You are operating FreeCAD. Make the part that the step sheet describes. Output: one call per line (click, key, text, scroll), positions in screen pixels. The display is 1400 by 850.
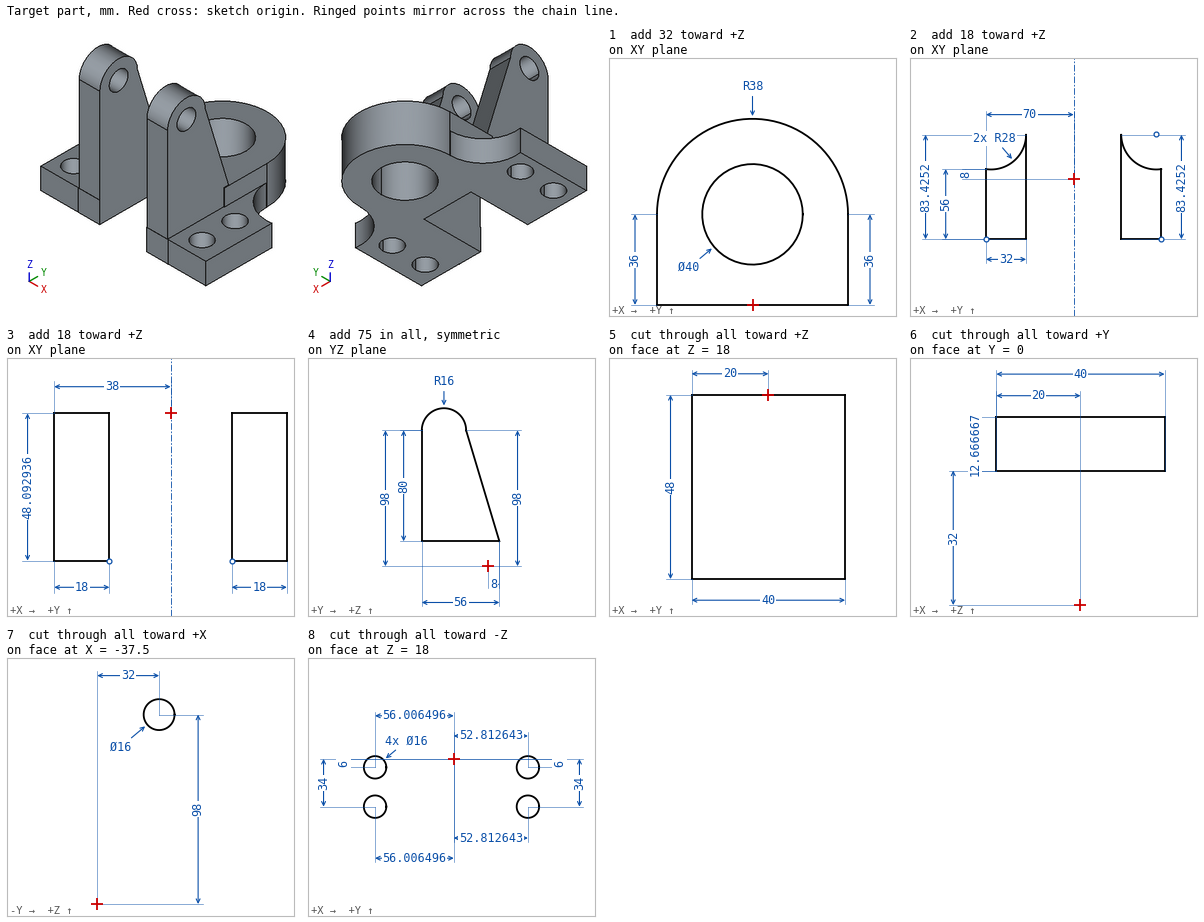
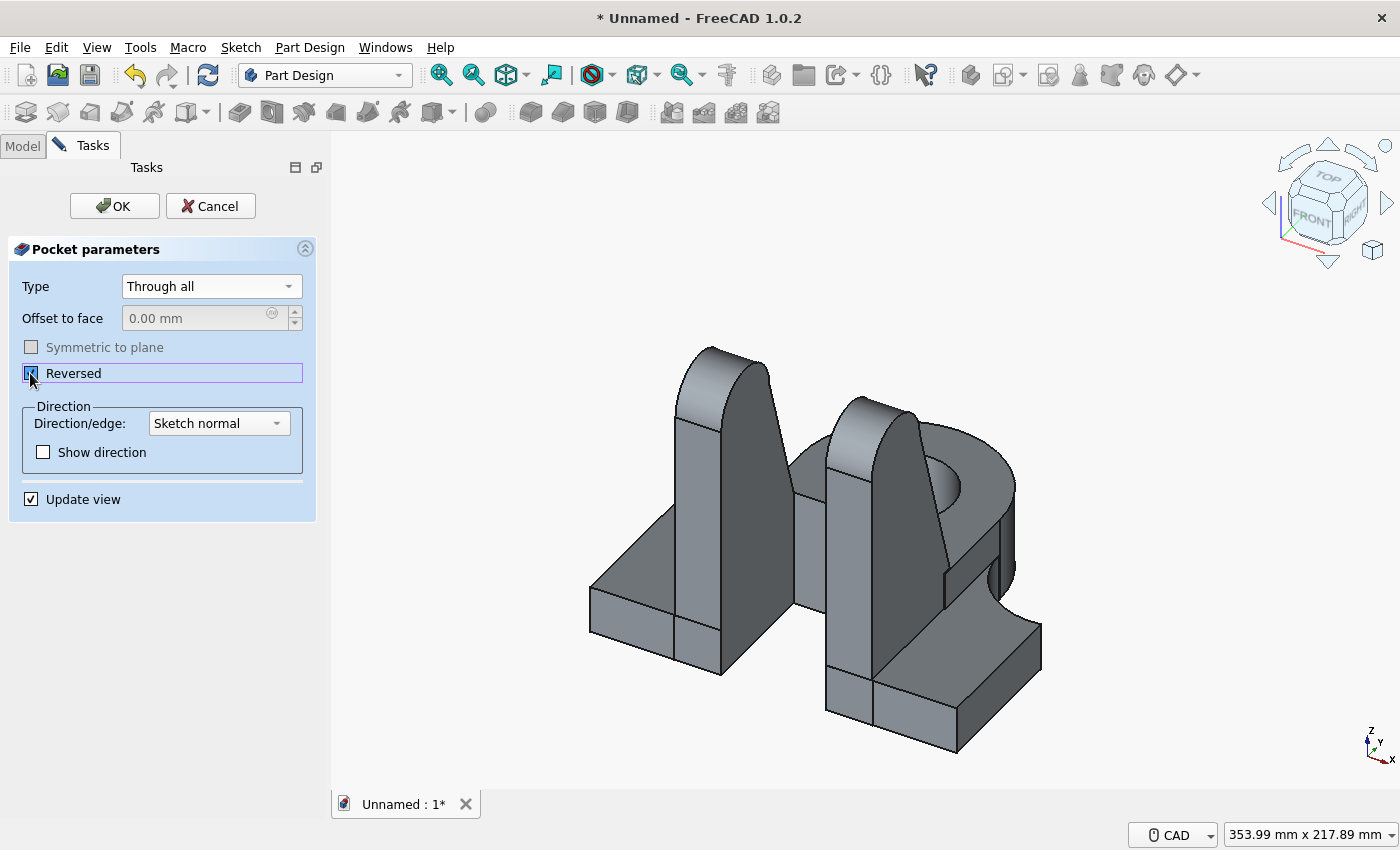
click(115, 206)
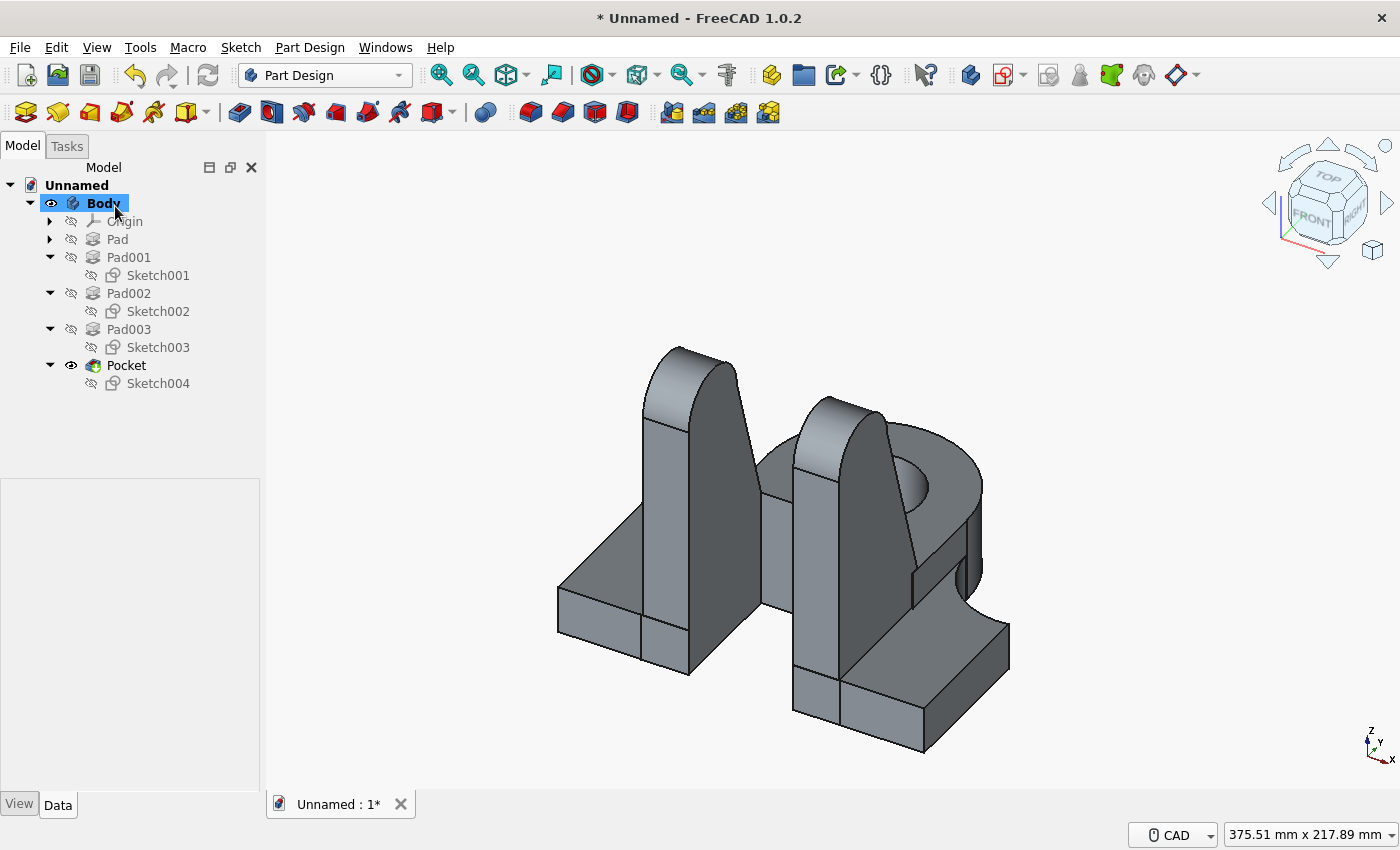
key(0)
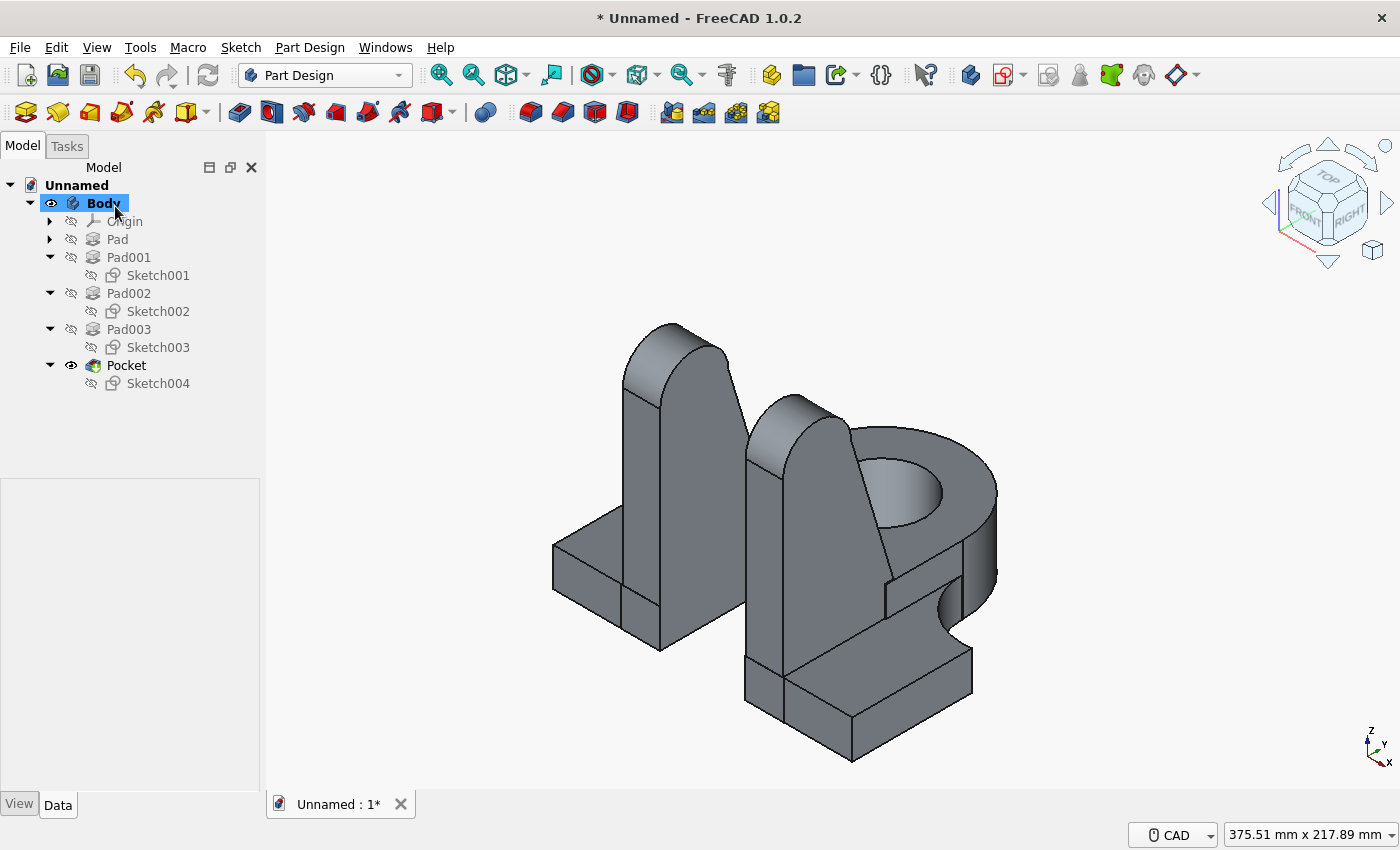
key(1)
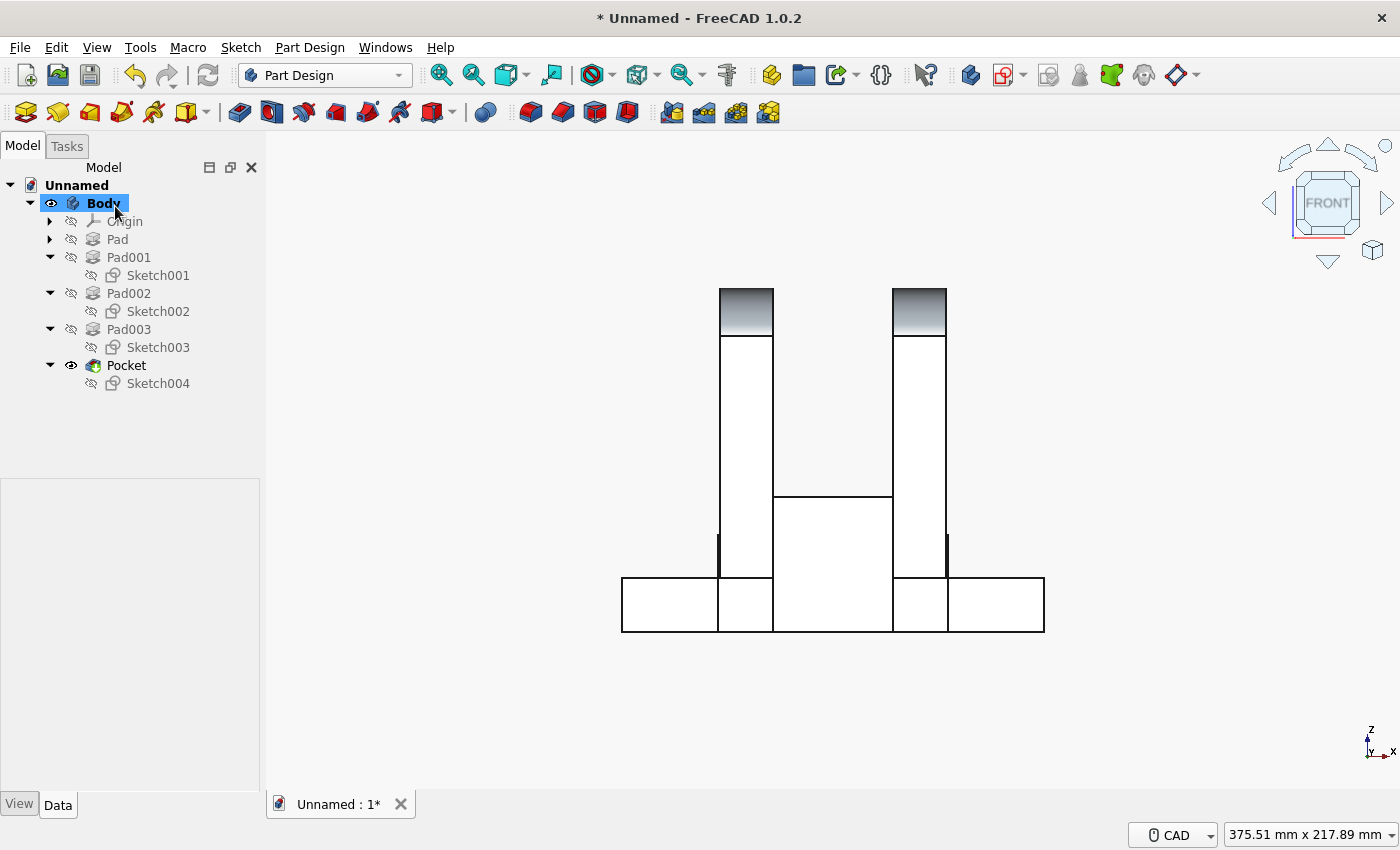
click(833, 564)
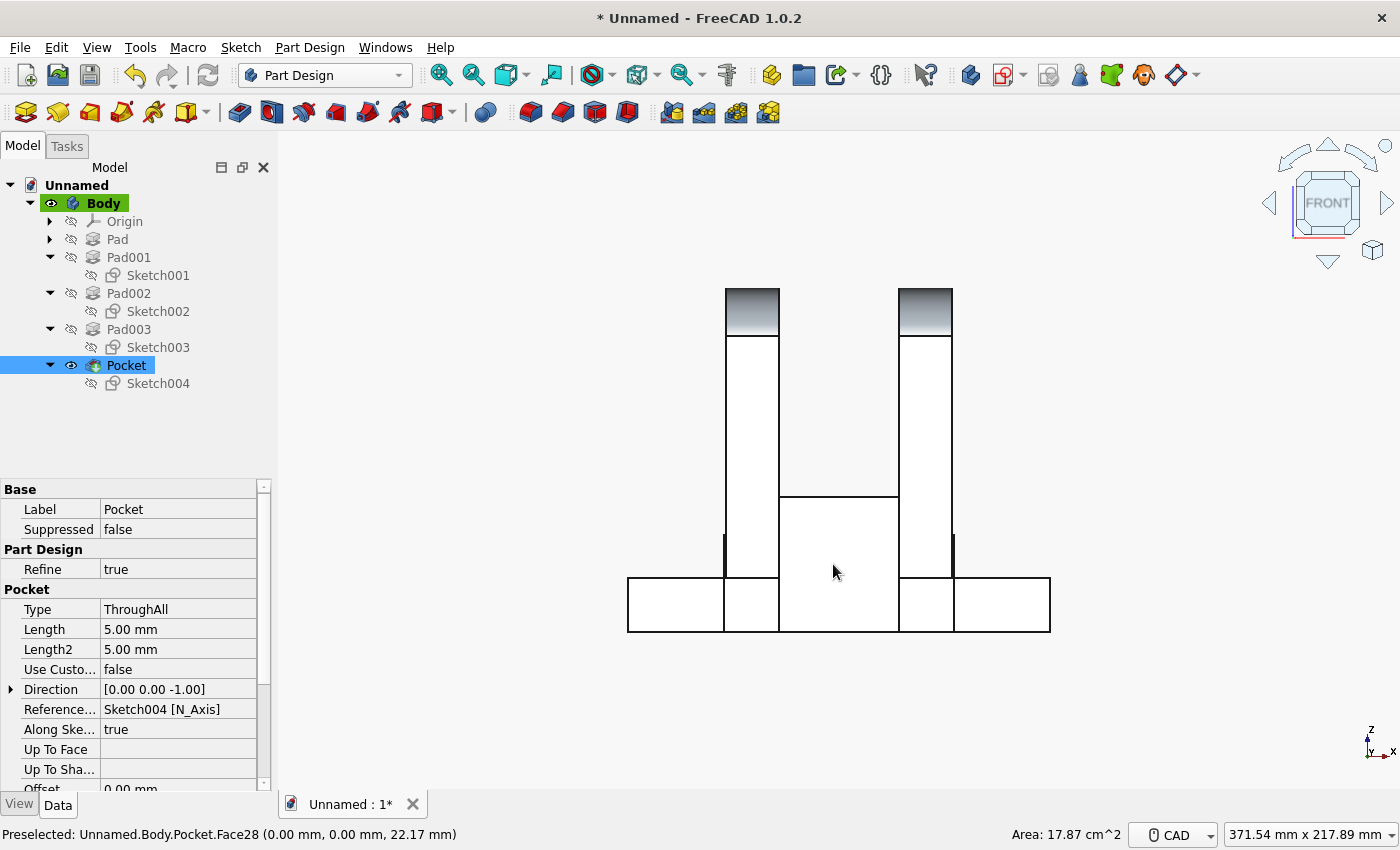
click(1004, 76)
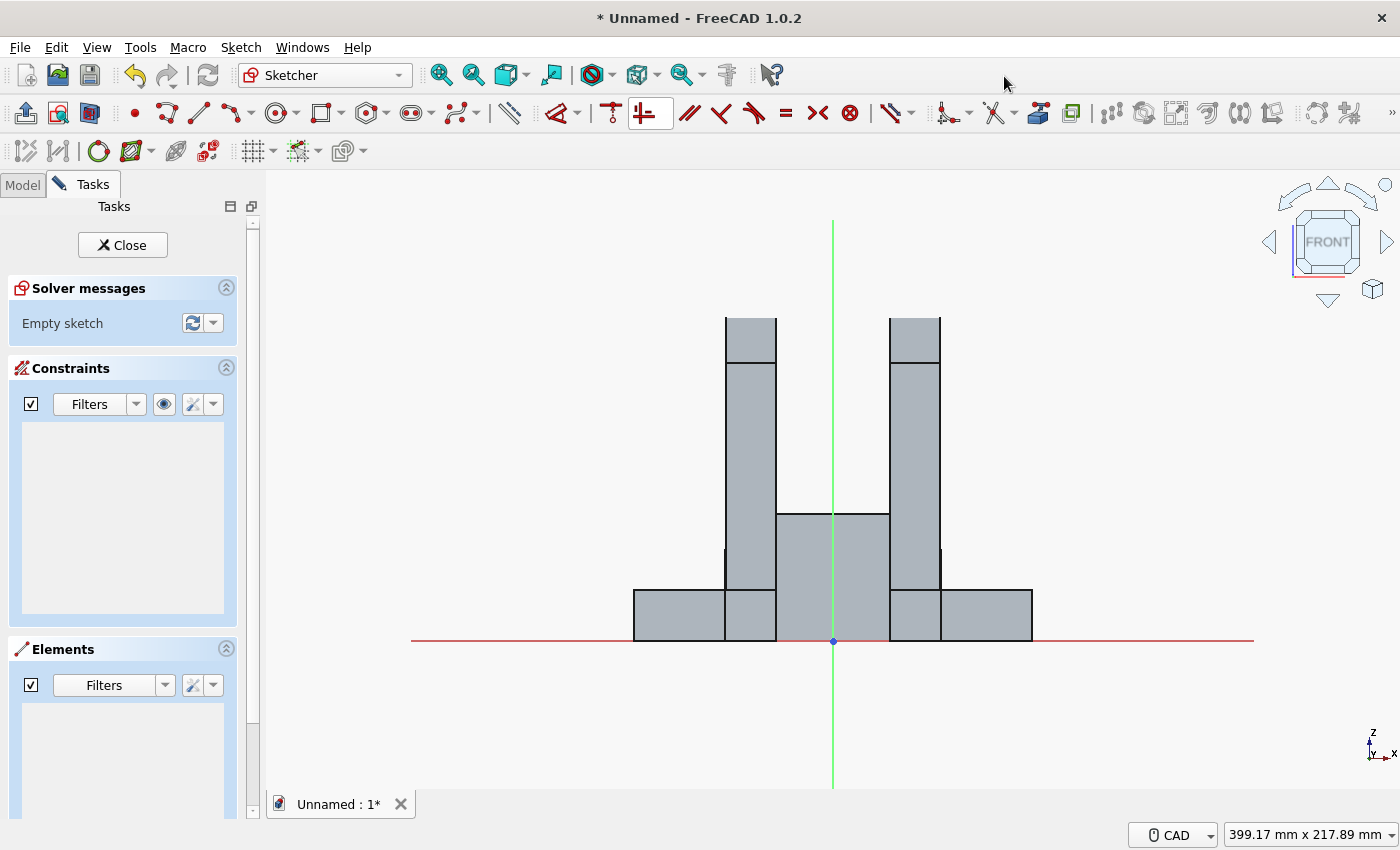
click(90, 114)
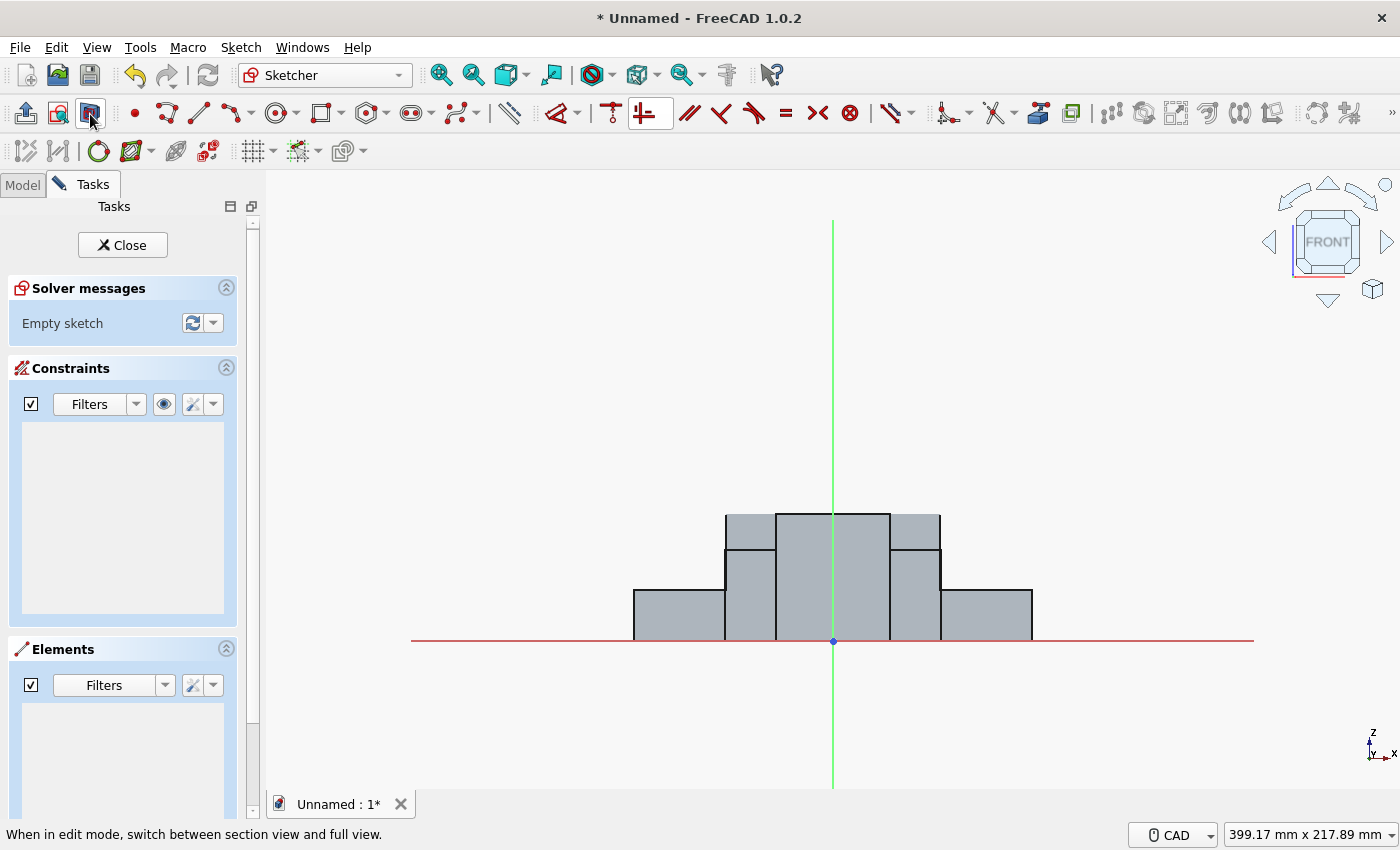
scroll(863, 620, up, 6)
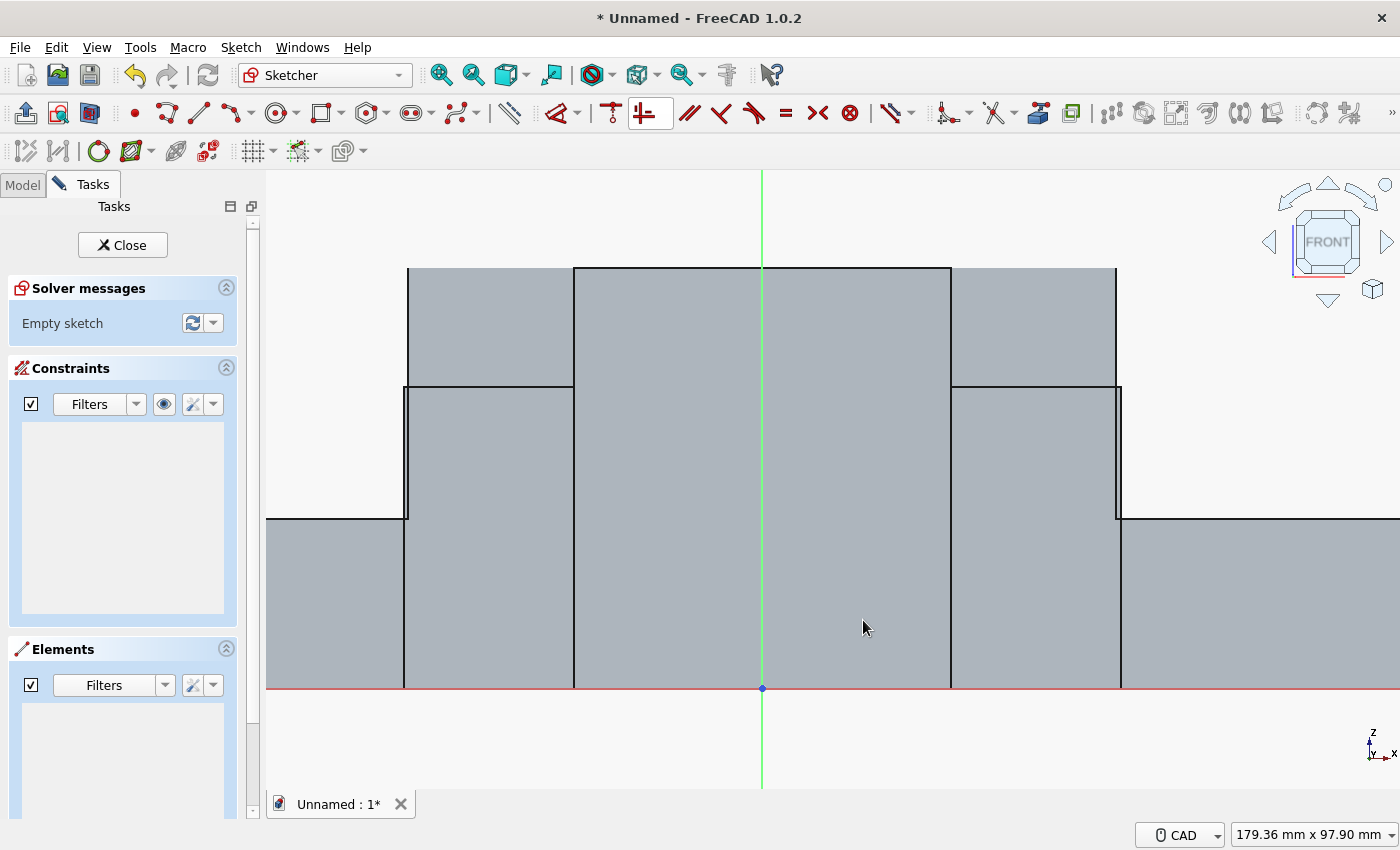
click(322, 114)